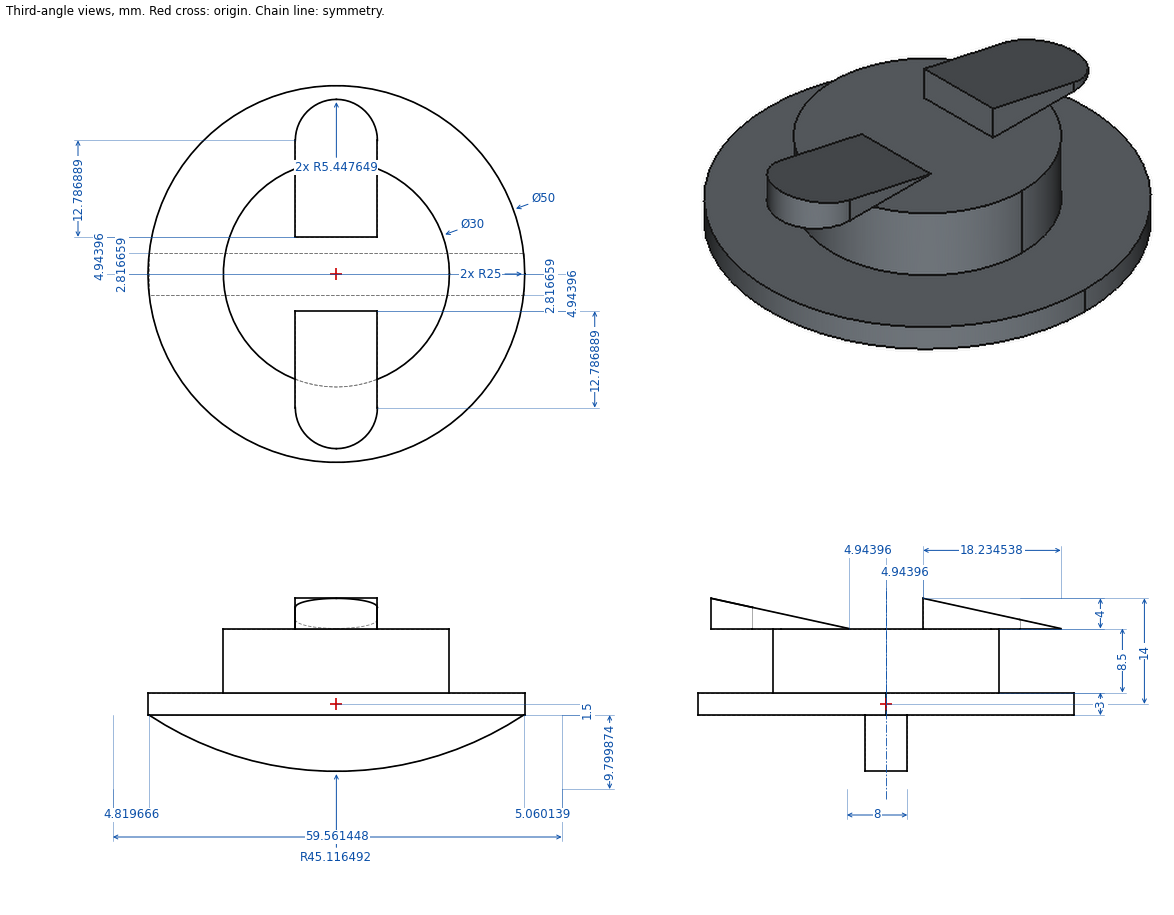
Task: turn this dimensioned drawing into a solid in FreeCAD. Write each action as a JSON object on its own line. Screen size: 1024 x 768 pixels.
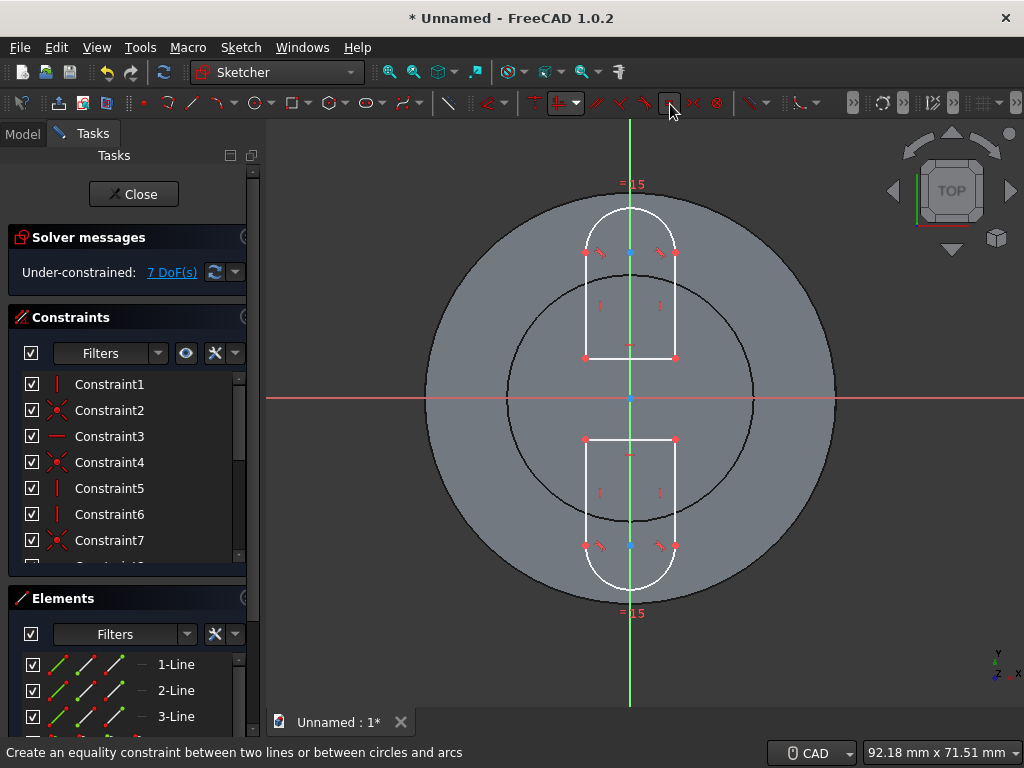
{"action": "left_click", "coordinate": [631, 253]}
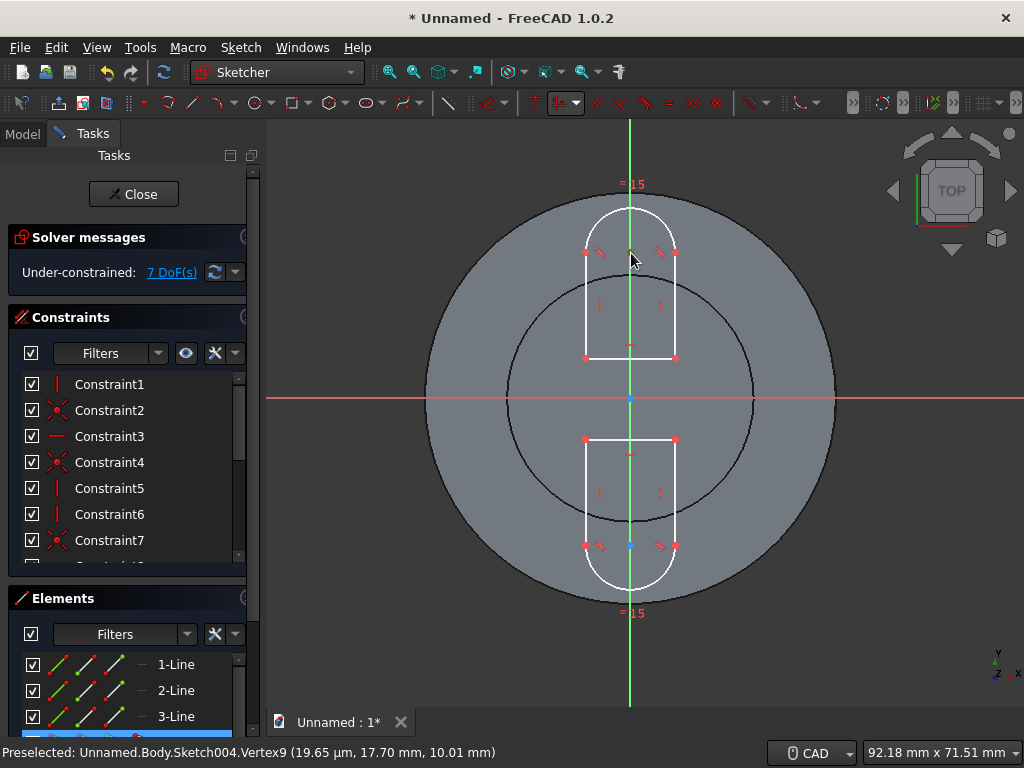
{"action": "left_click", "coordinate": [630, 641]}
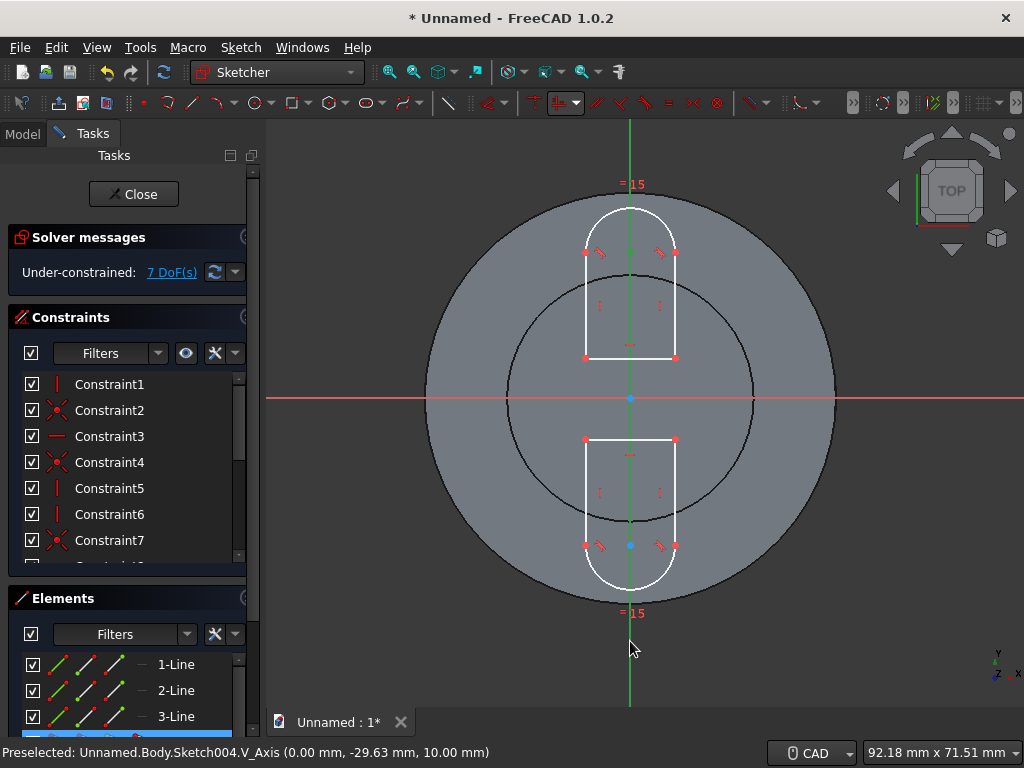
{"action": "left_click", "coordinate": [534, 104]}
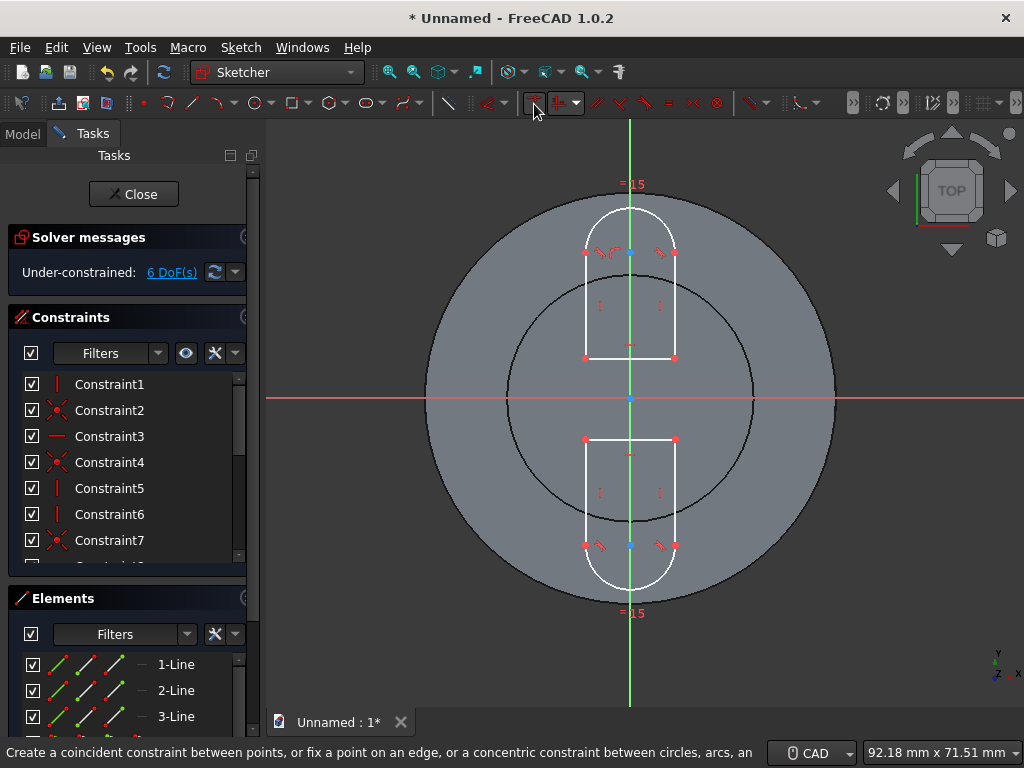
{"action": "left_click", "coordinate": [630, 545]}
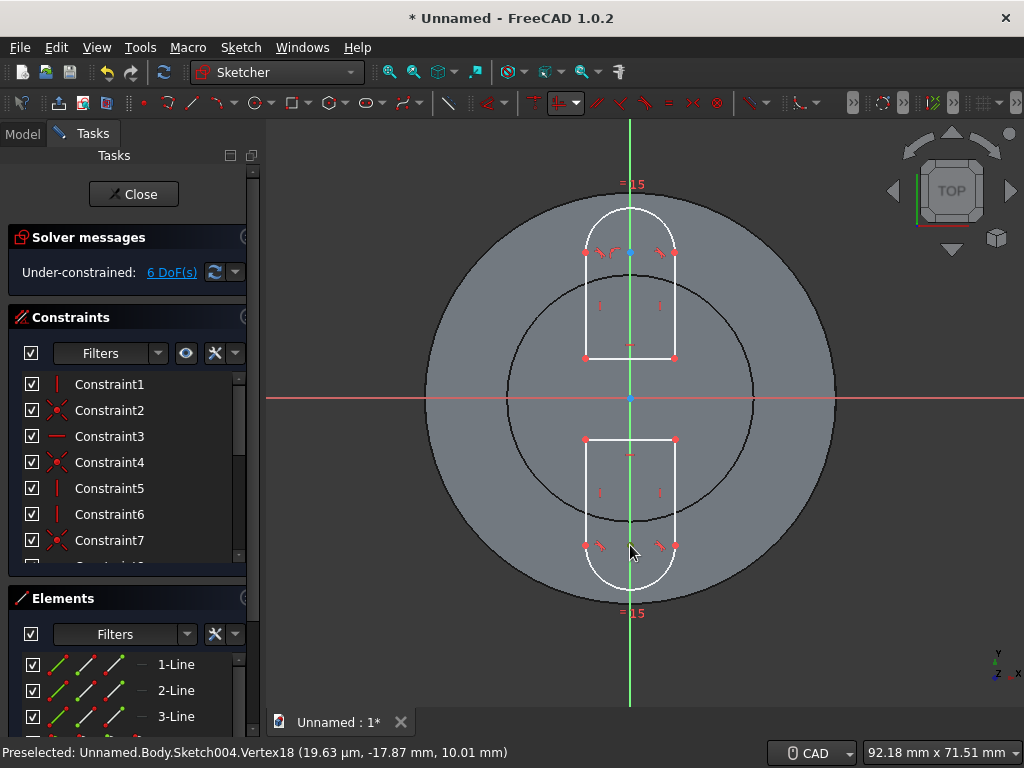
{"action": "left_click", "coordinate": [630, 641]}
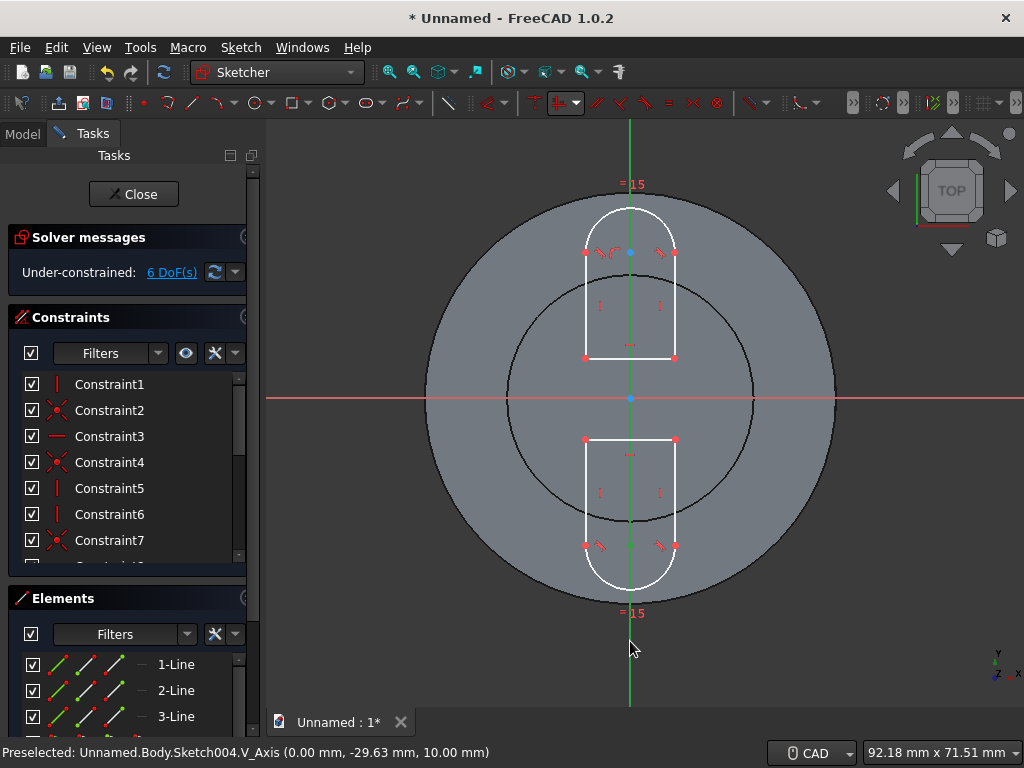
{"action": "key", "text": "c"}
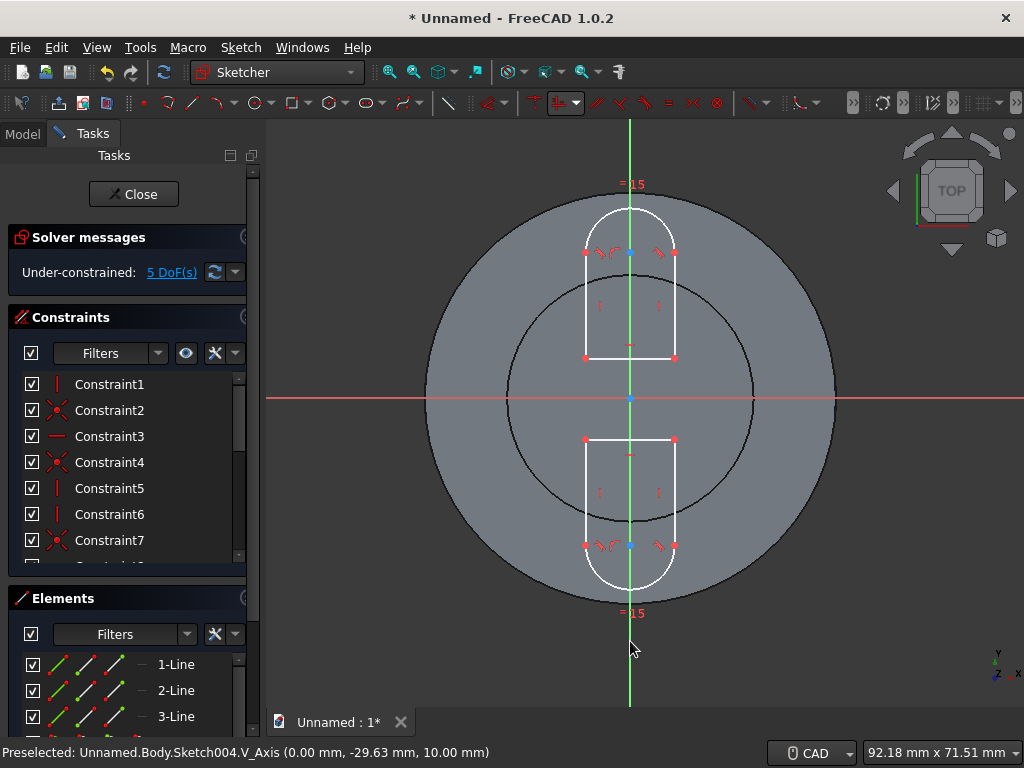
{"action": "left_click", "coordinate": [488, 104]}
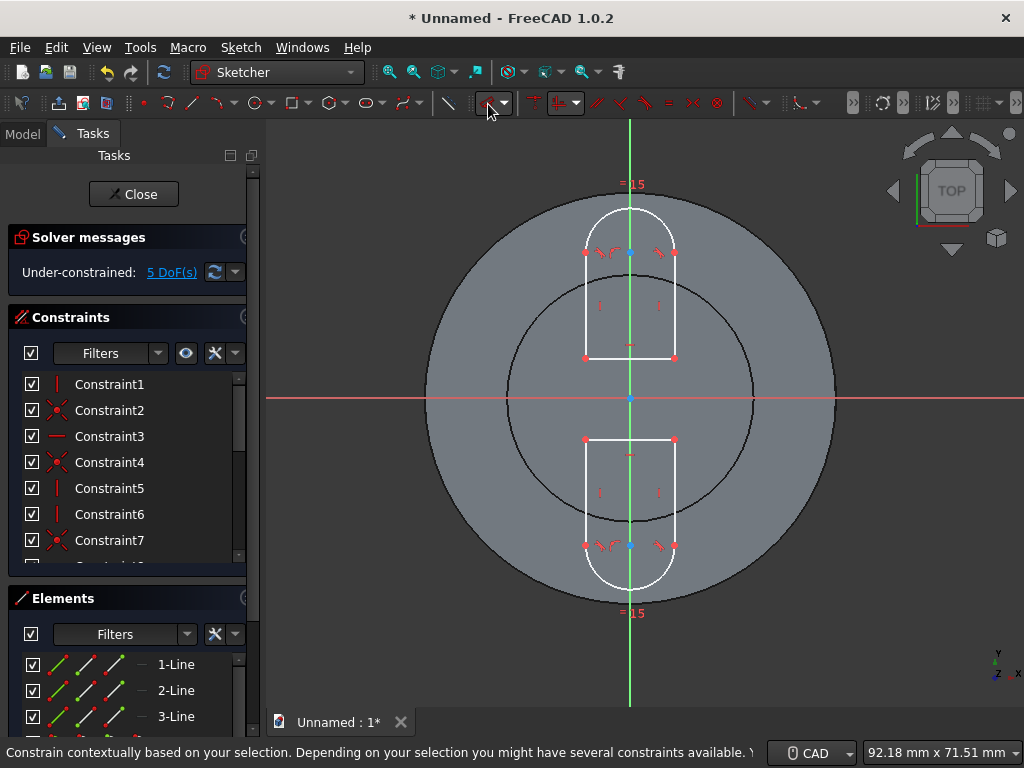
{"action": "left_click", "coordinate": [656, 217]}
{"action": "left_click", "coordinate": [675, 191]}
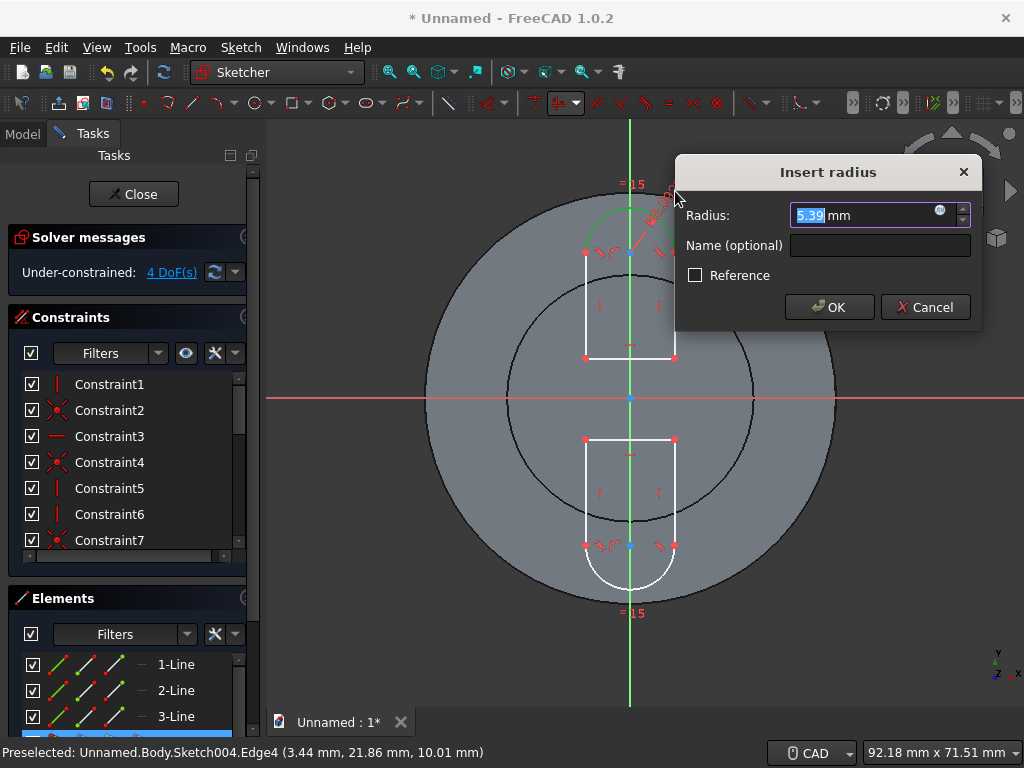
{"action": "type", "text": "5.447649"}
{"action": "key", "text": "Return"}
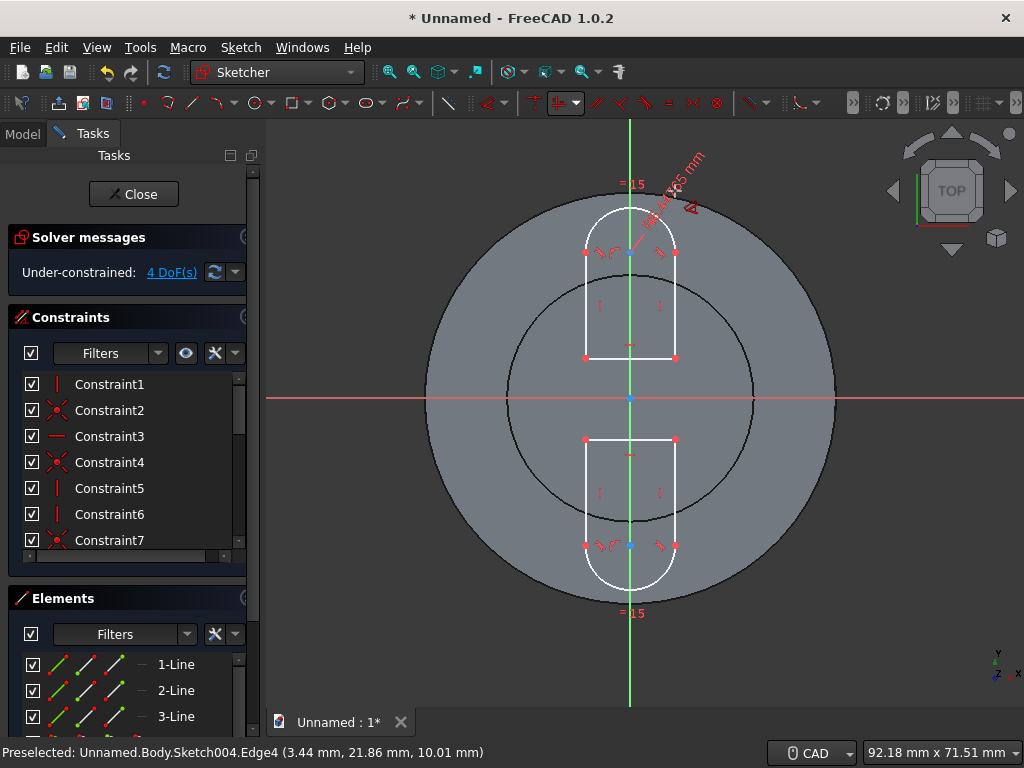
{"action": "left_click", "coordinate": [586, 359]}
{"action": "left_click", "coordinate": [552, 379]}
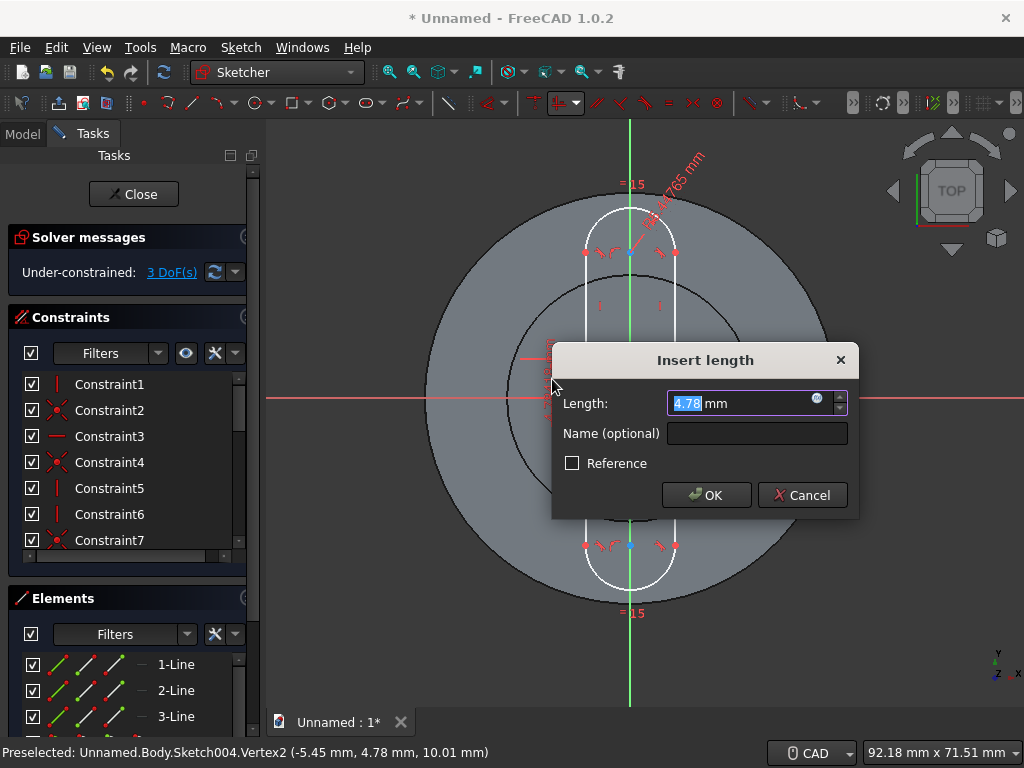
{"action": "type", "text": "4.94396"}
{"action": "key", "text": "Return"}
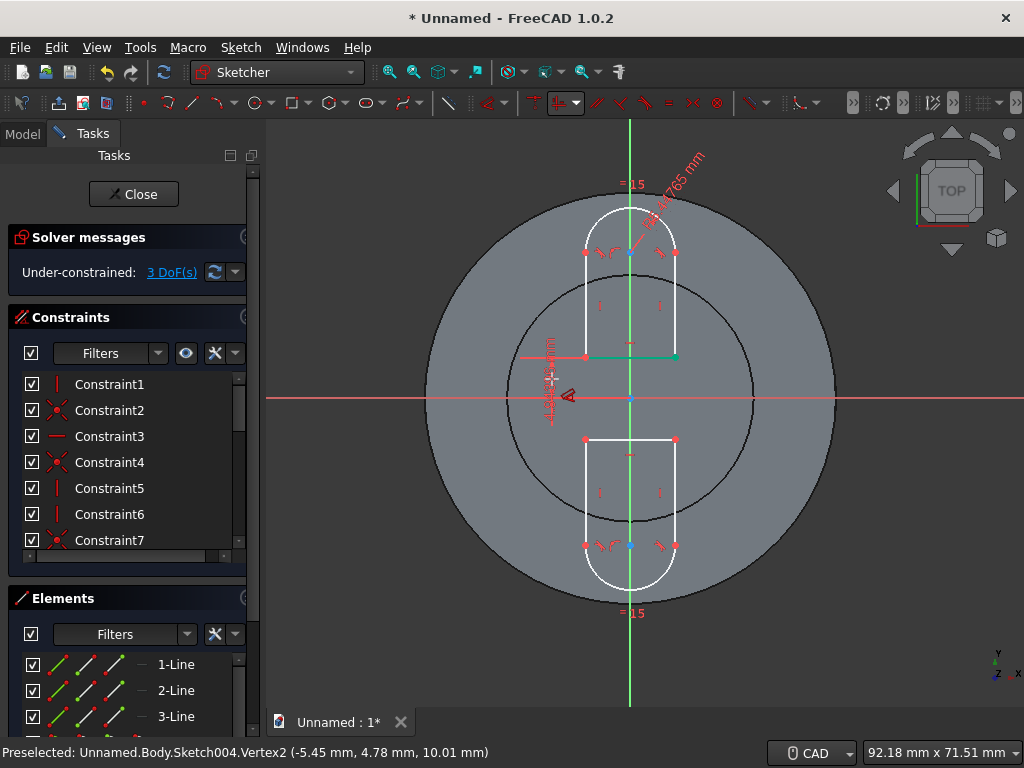
{"action": "left_click", "coordinate": [675, 440]}
{"action": "left_click", "coordinate": [709, 419]}